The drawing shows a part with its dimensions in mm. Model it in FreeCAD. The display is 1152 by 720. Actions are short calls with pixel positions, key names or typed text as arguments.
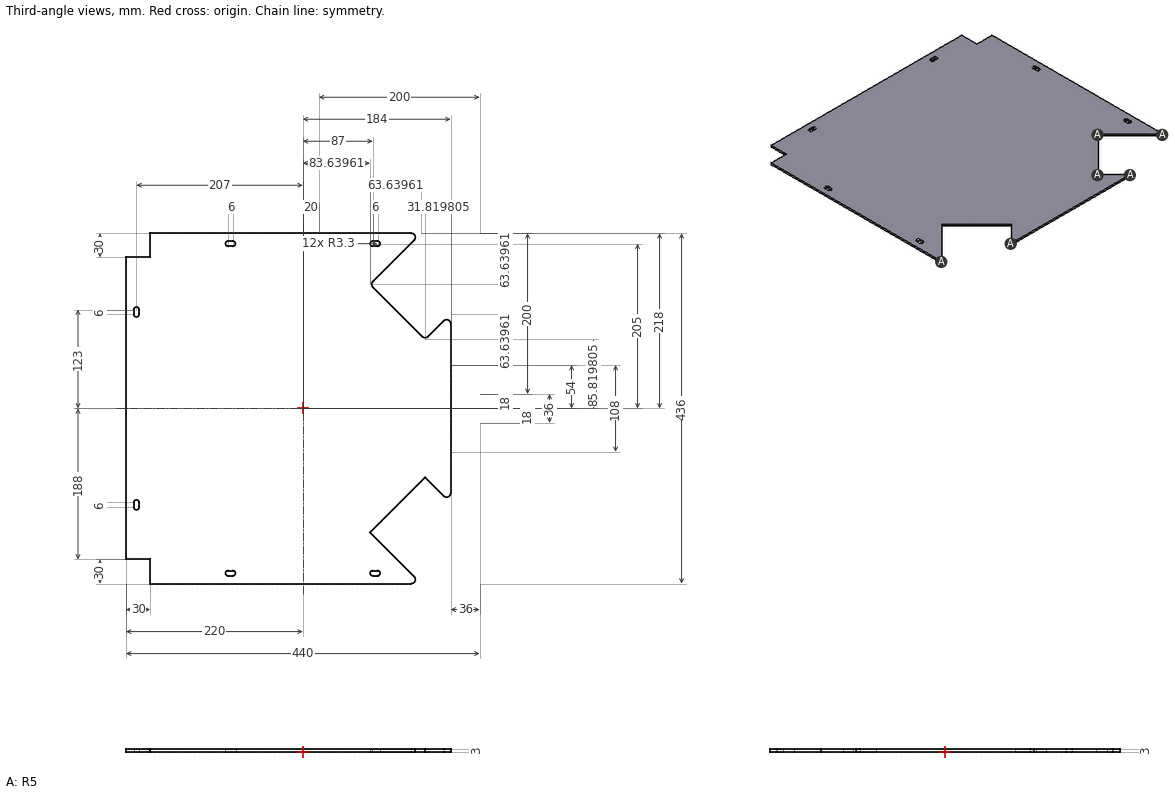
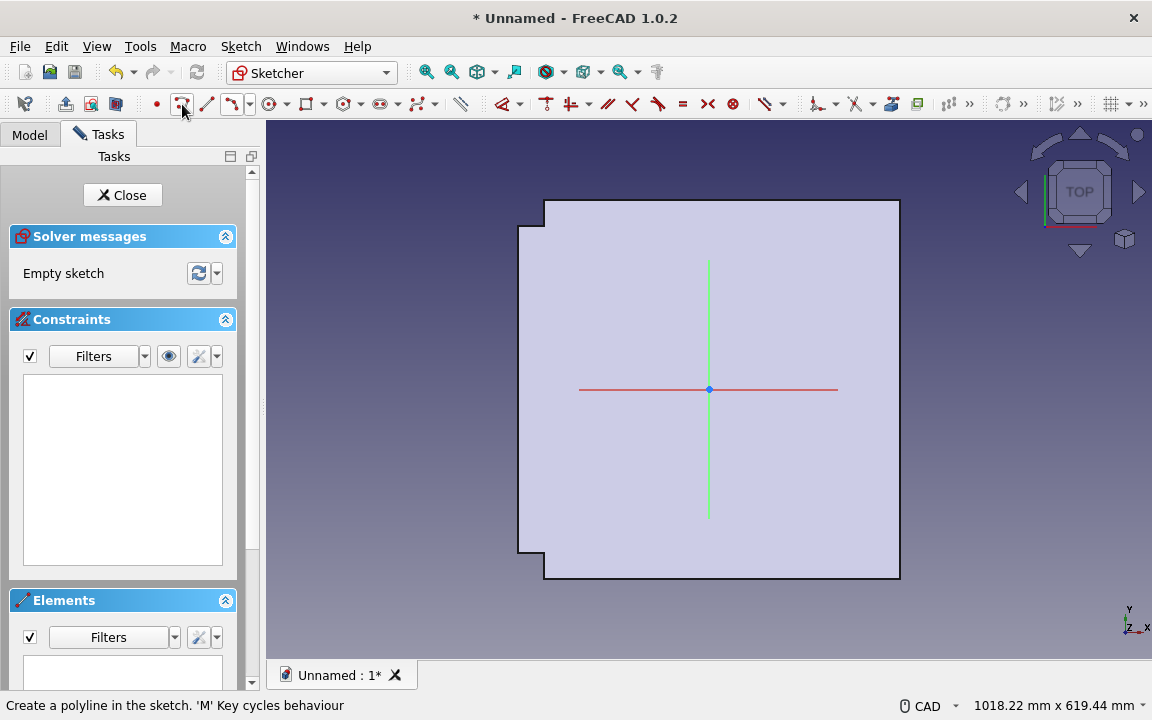
click(726, 200)
click(900, 374)
click(900, 200)
click(726, 201)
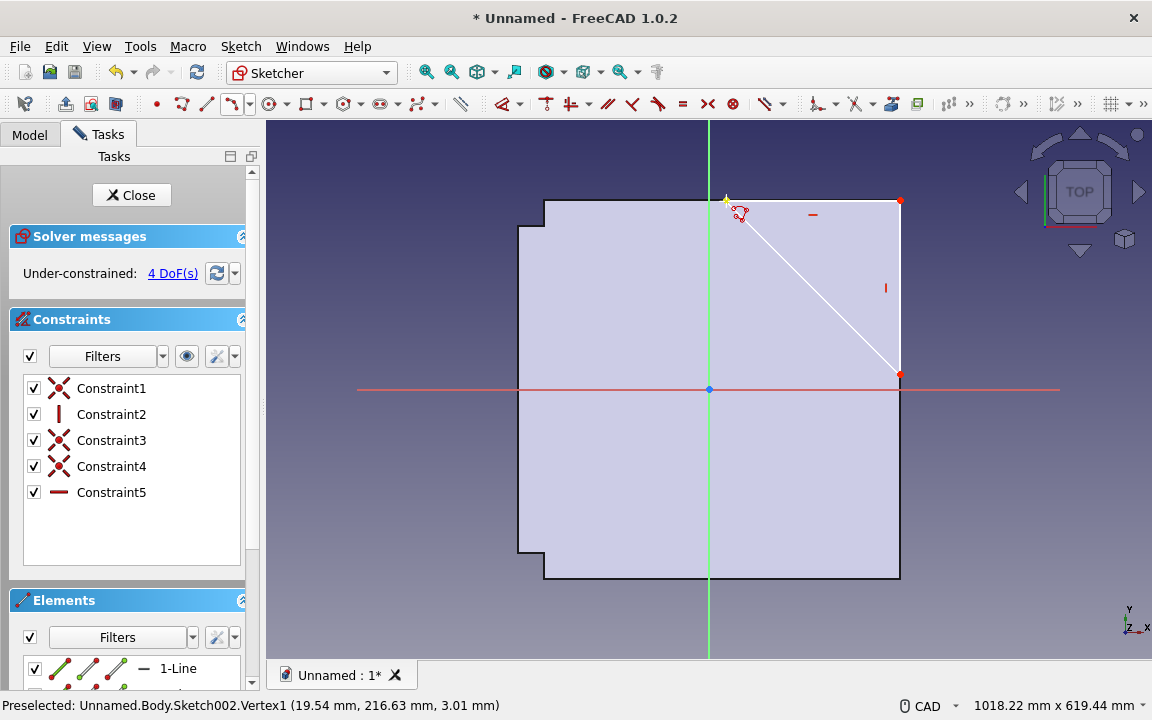
click(726, 579)
click(900, 579)
click(900, 405)
click(726, 580)
key(Escape)
key(Escape)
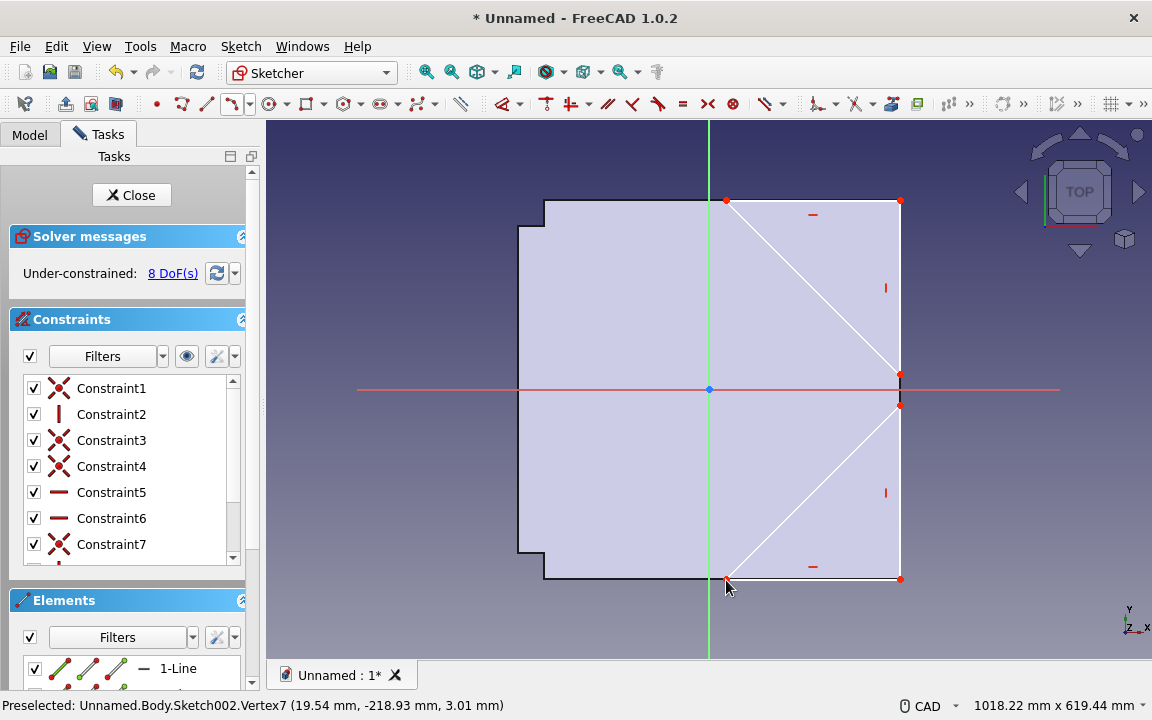
click(726, 201)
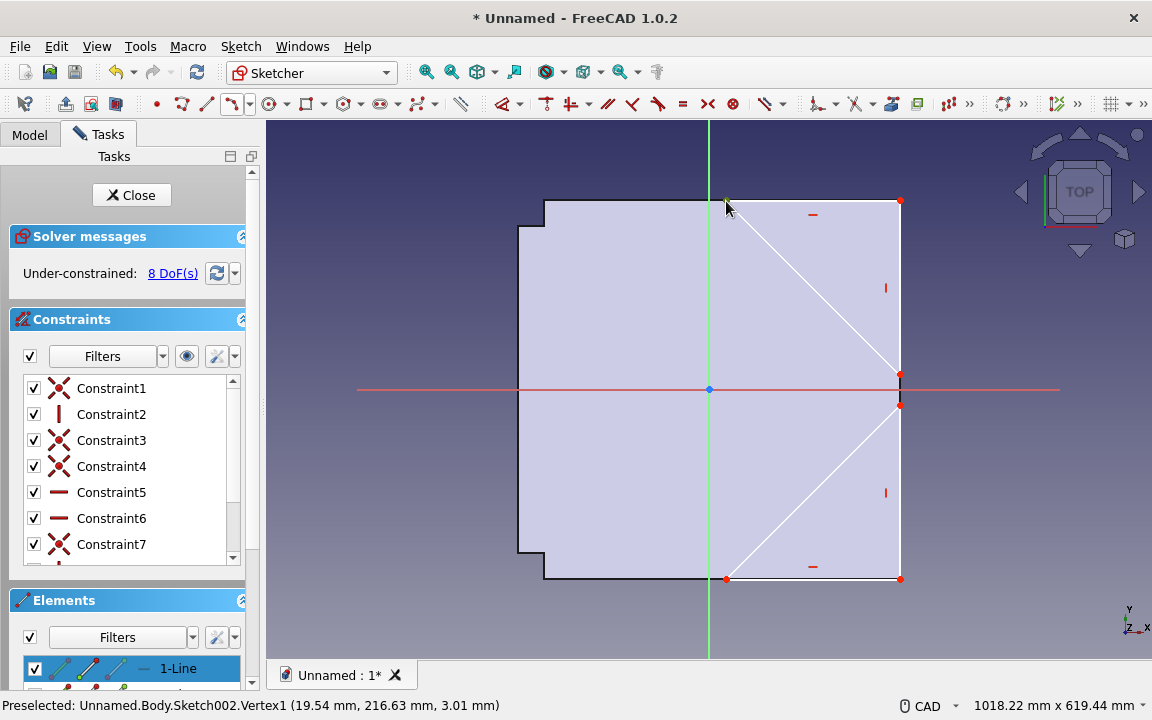
click(726, 580)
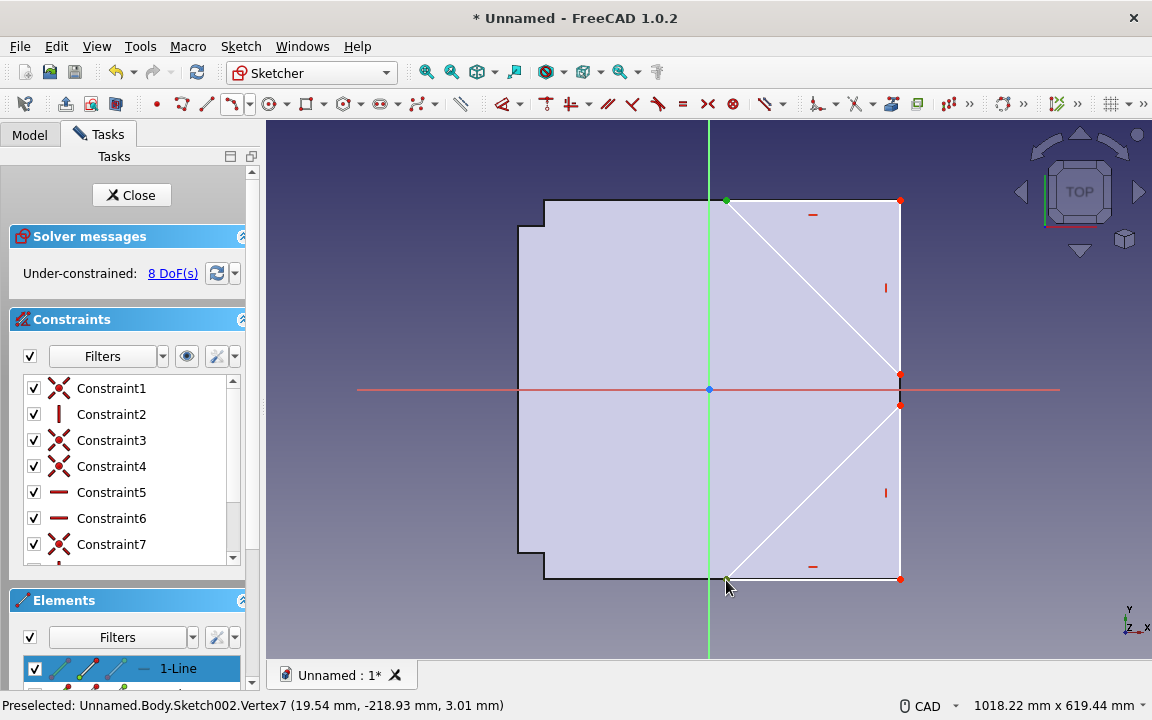
click(393, 390)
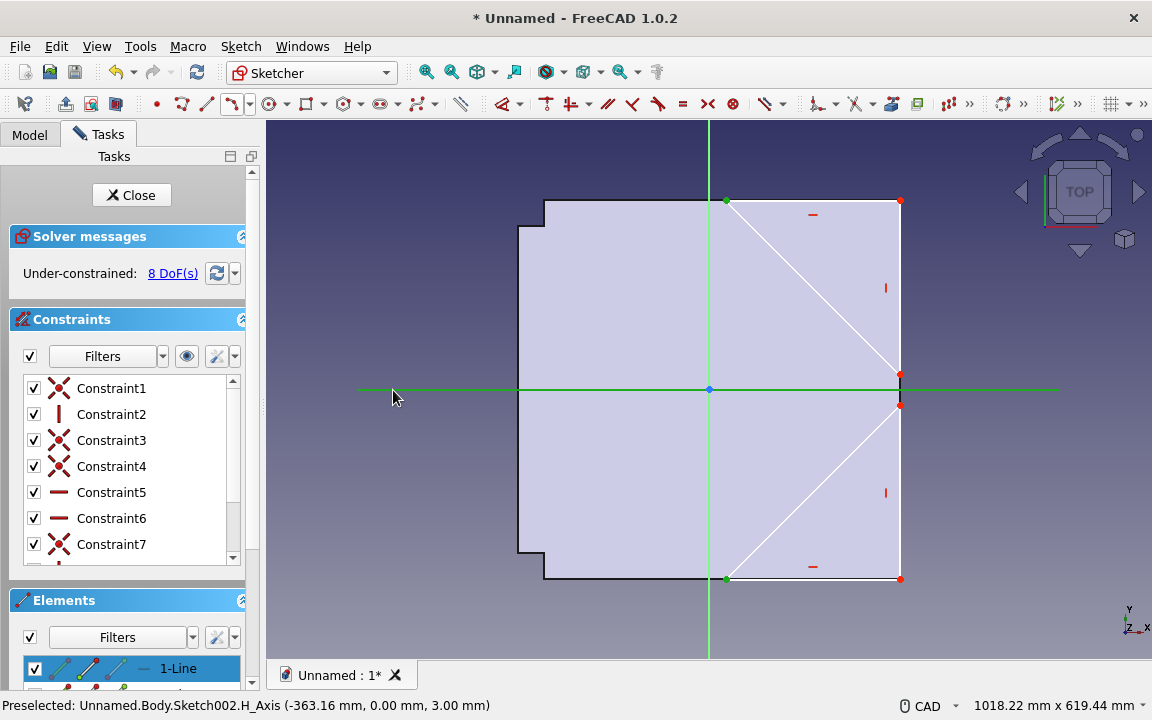
key(s)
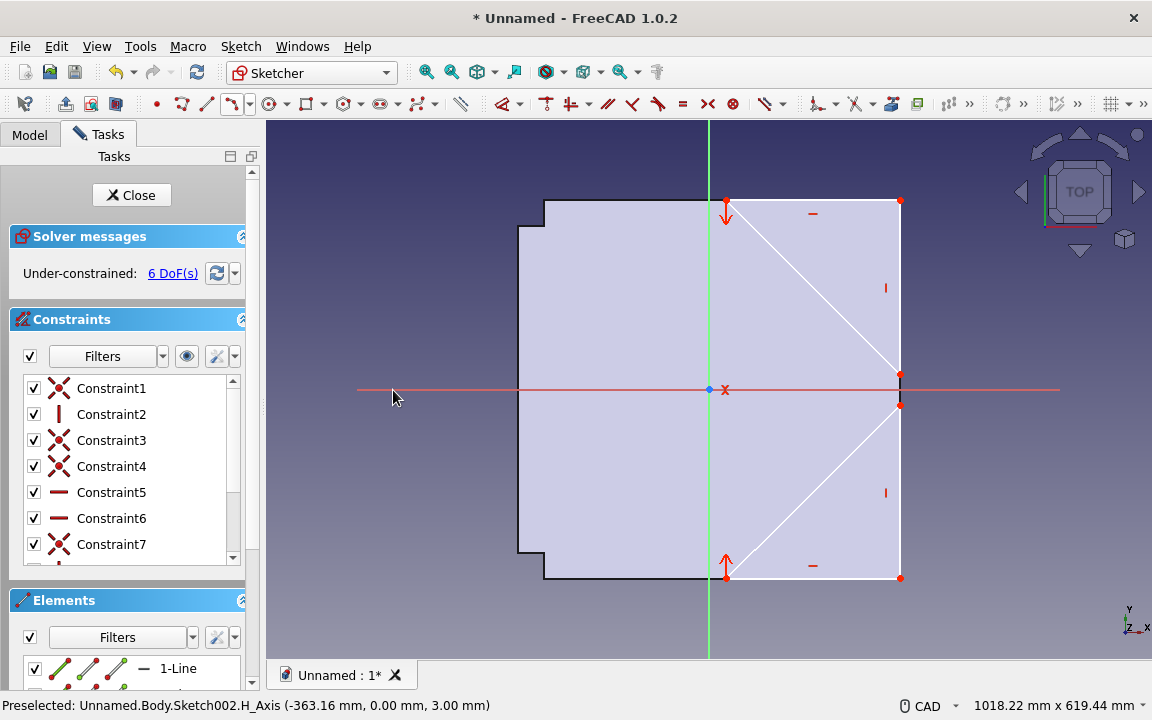
click(900, 375)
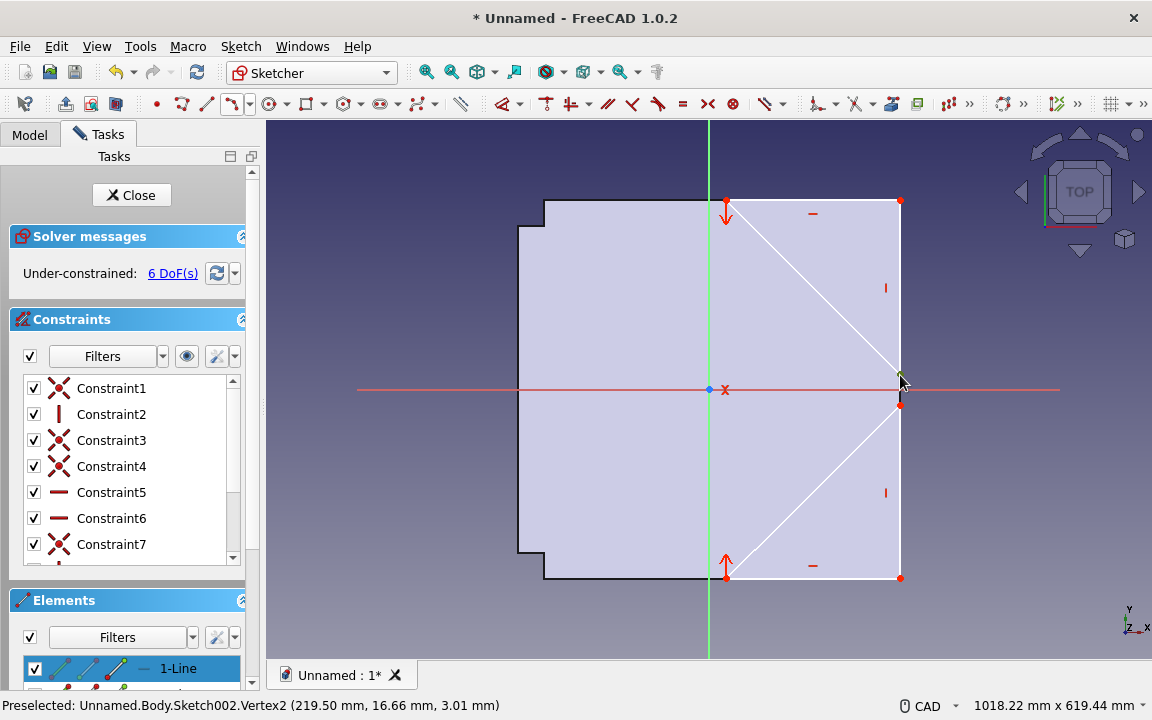
click(900, 406)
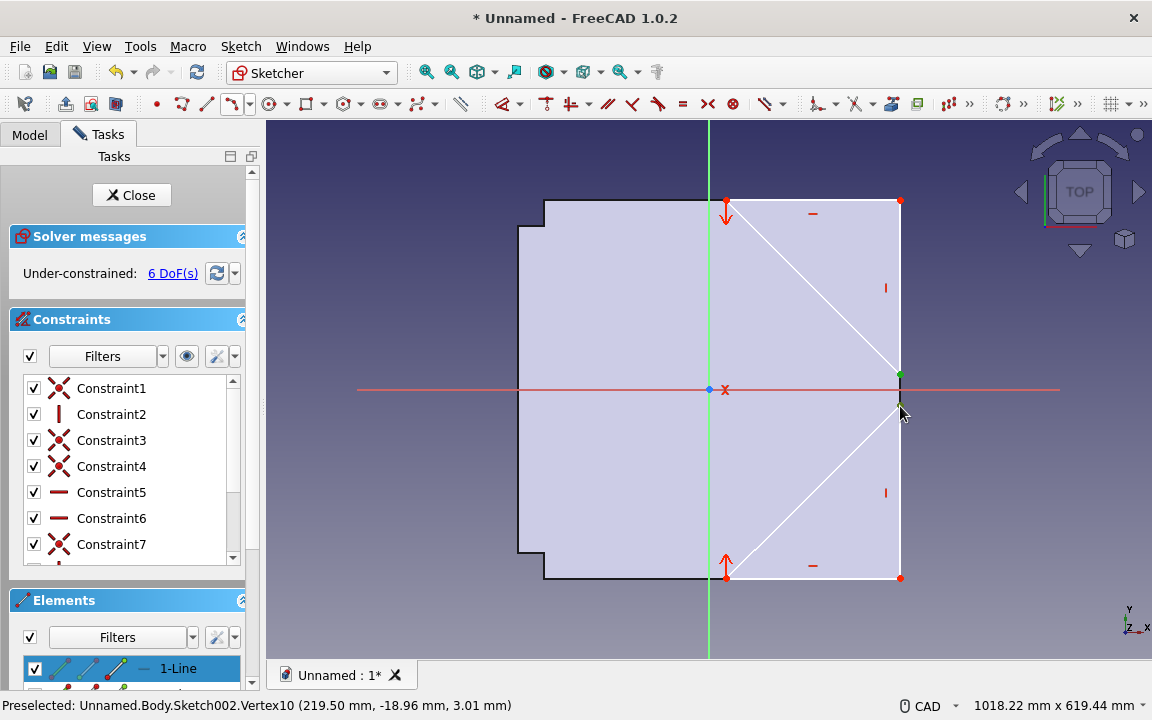
click(393, 390)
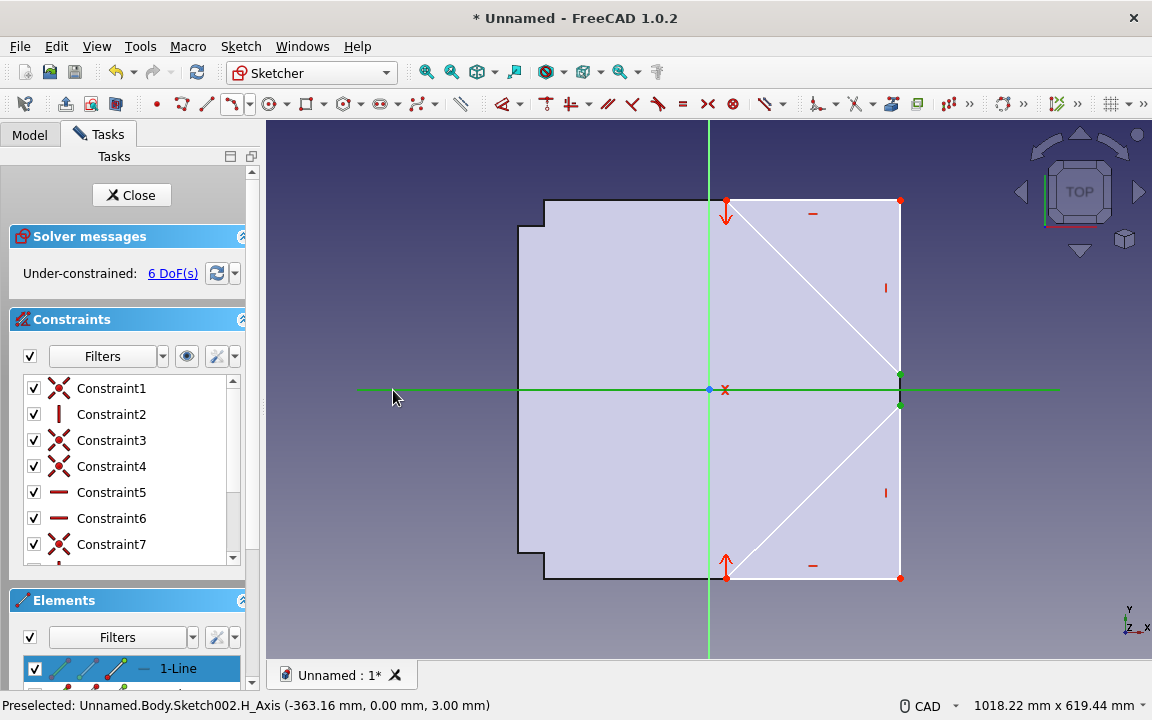
key(s)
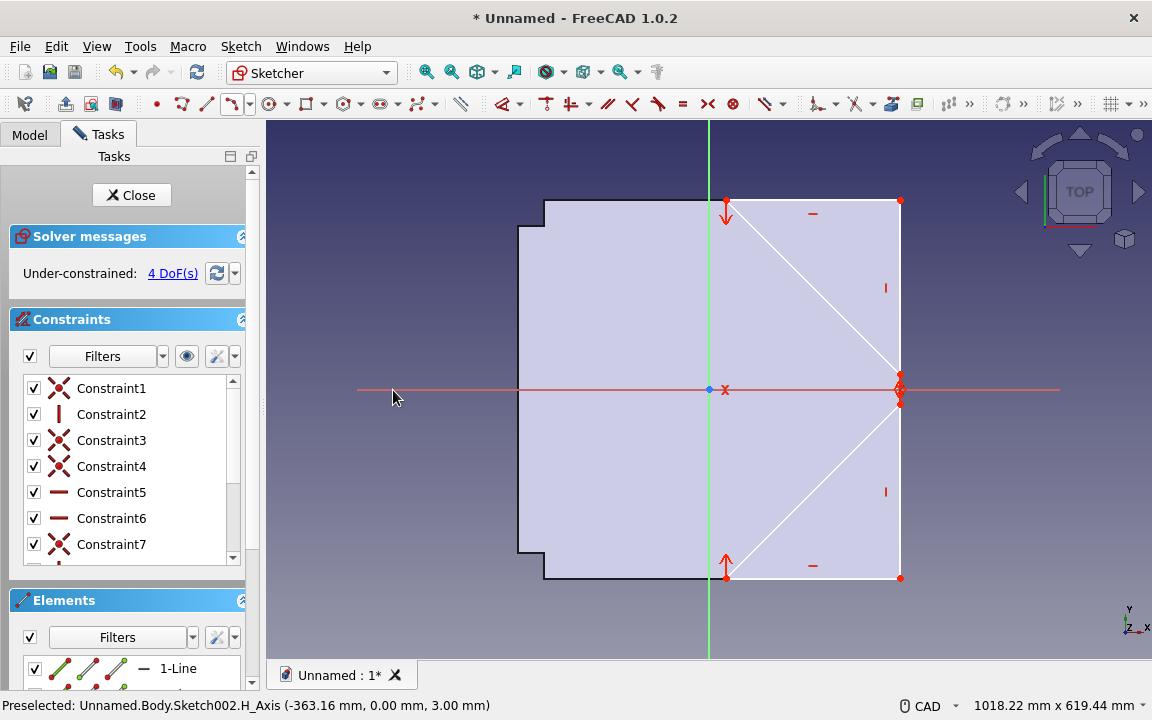
key(d)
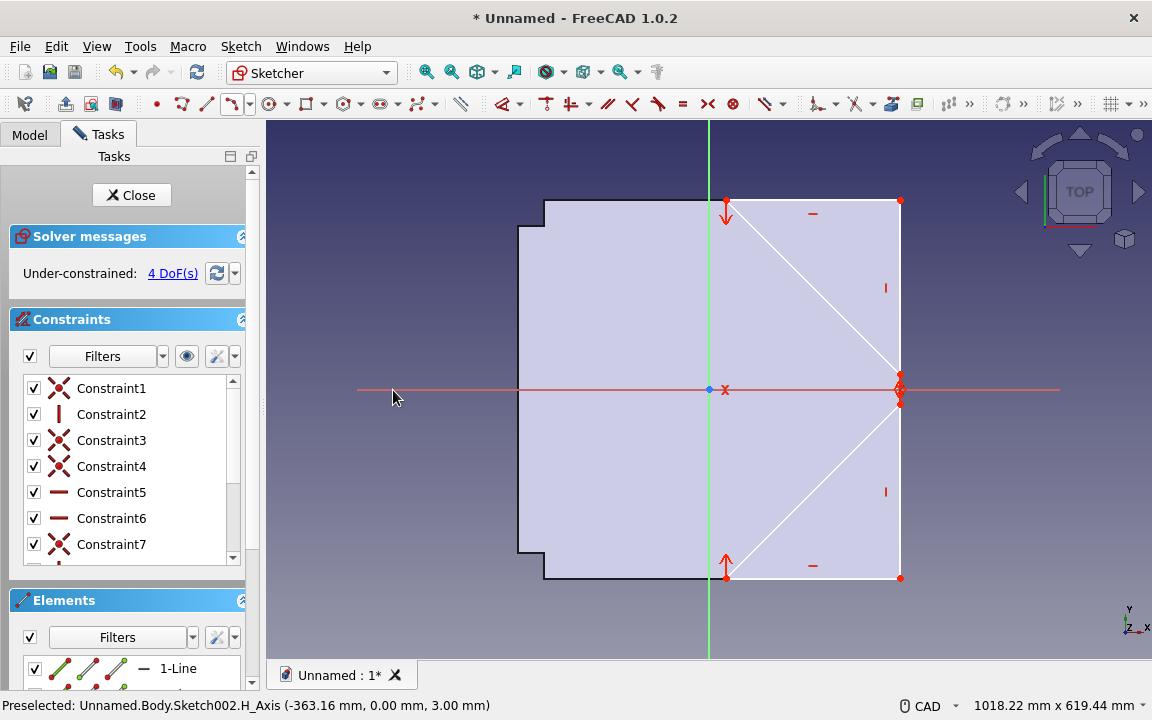
click(900, 322)
click(934, 287)